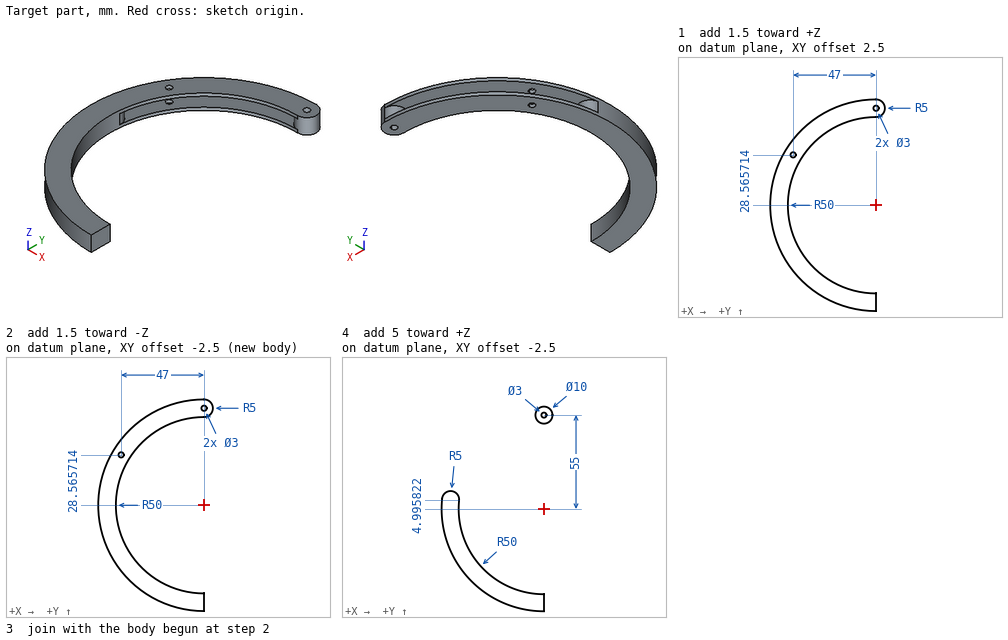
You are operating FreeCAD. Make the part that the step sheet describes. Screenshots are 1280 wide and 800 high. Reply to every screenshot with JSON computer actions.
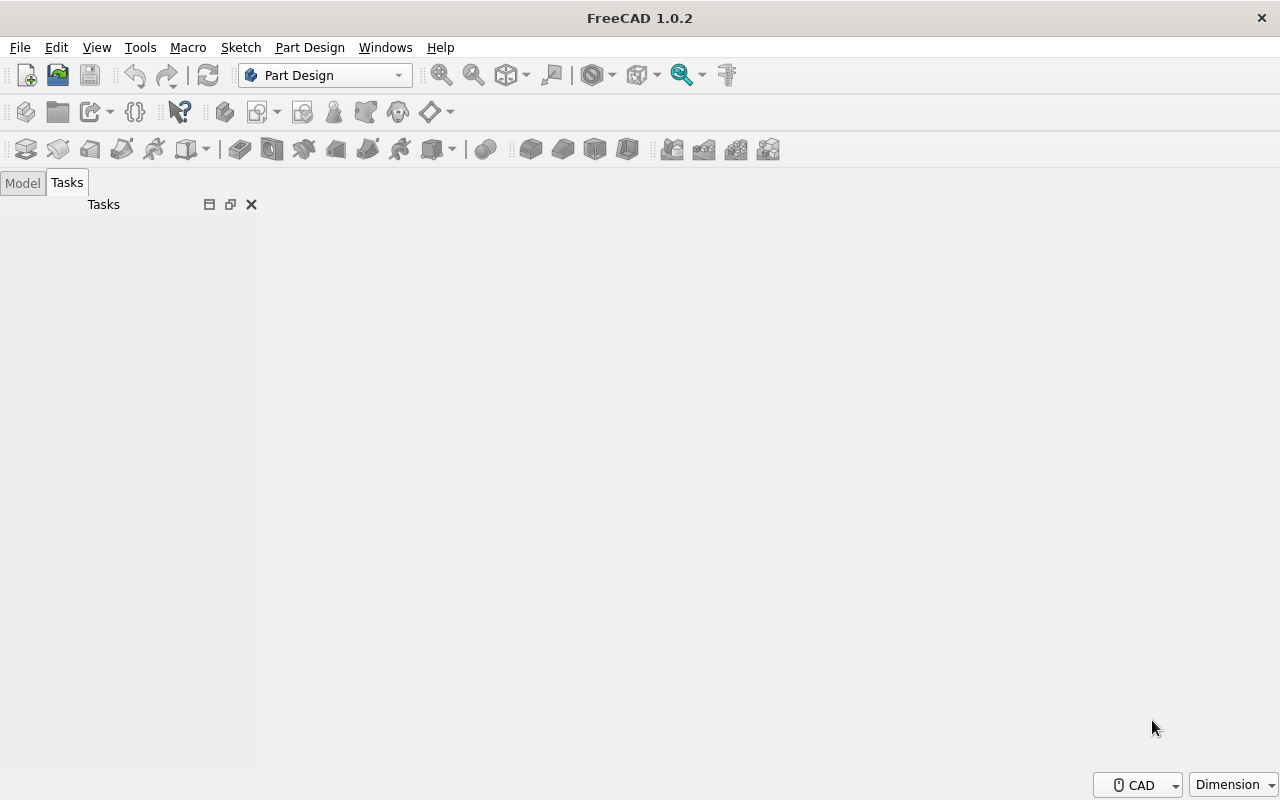
{"action": "left_click", "coordinate": [26, 76]}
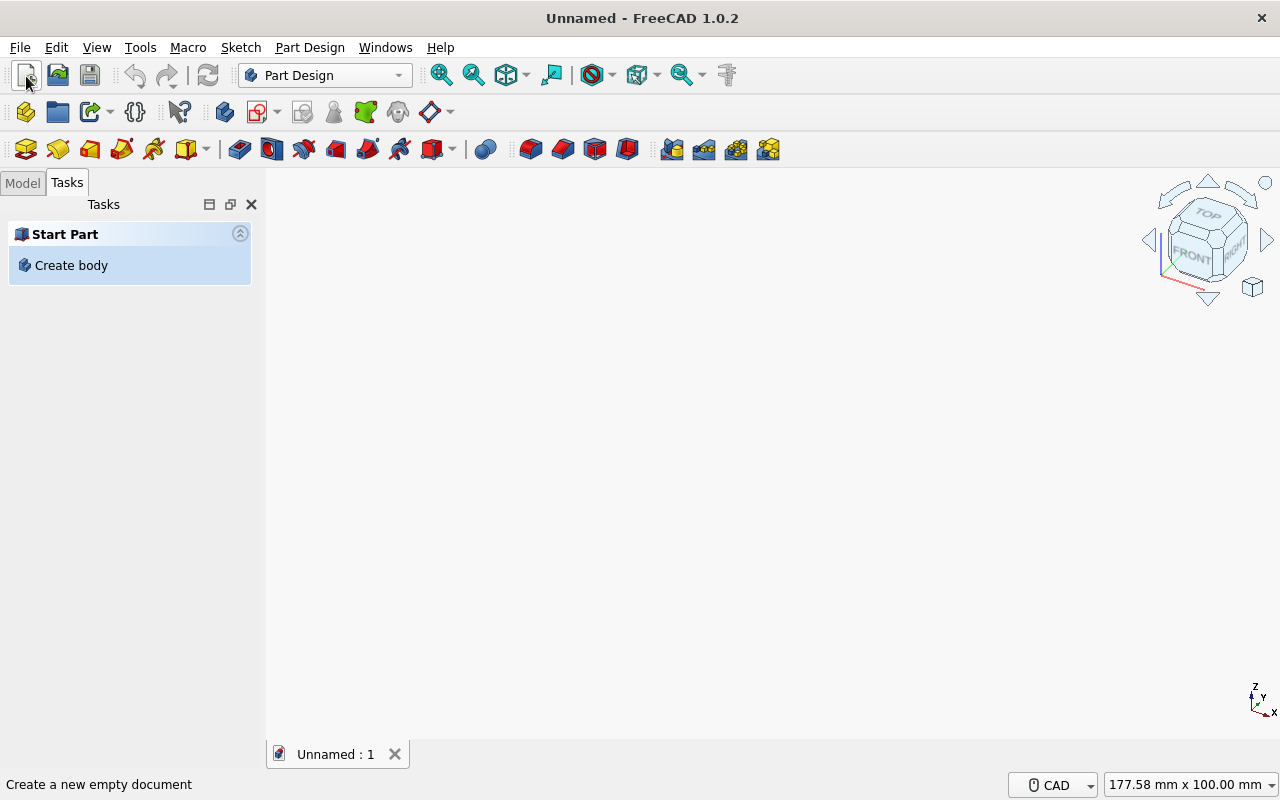
{"action": "left_click", "coordinate": [226, 112]}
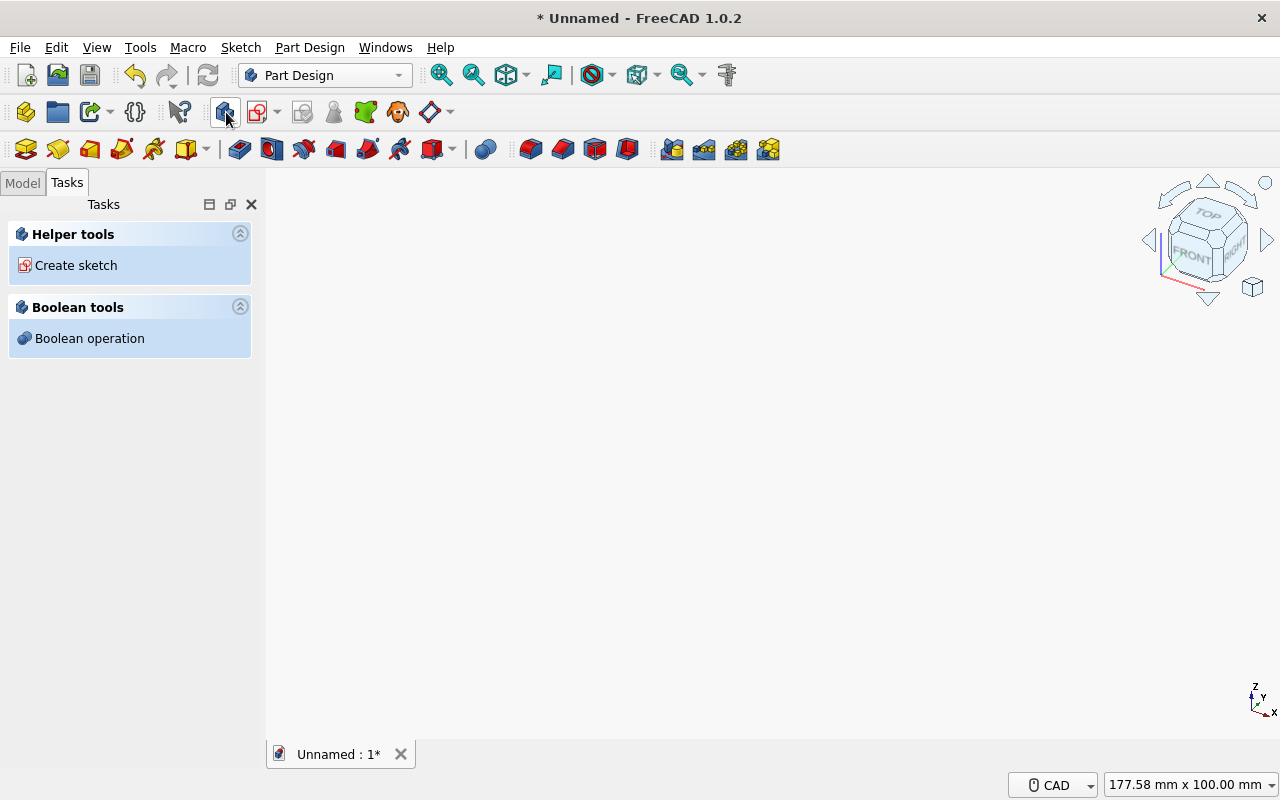
{"action": "left_click", "coordinate": [23, 182]}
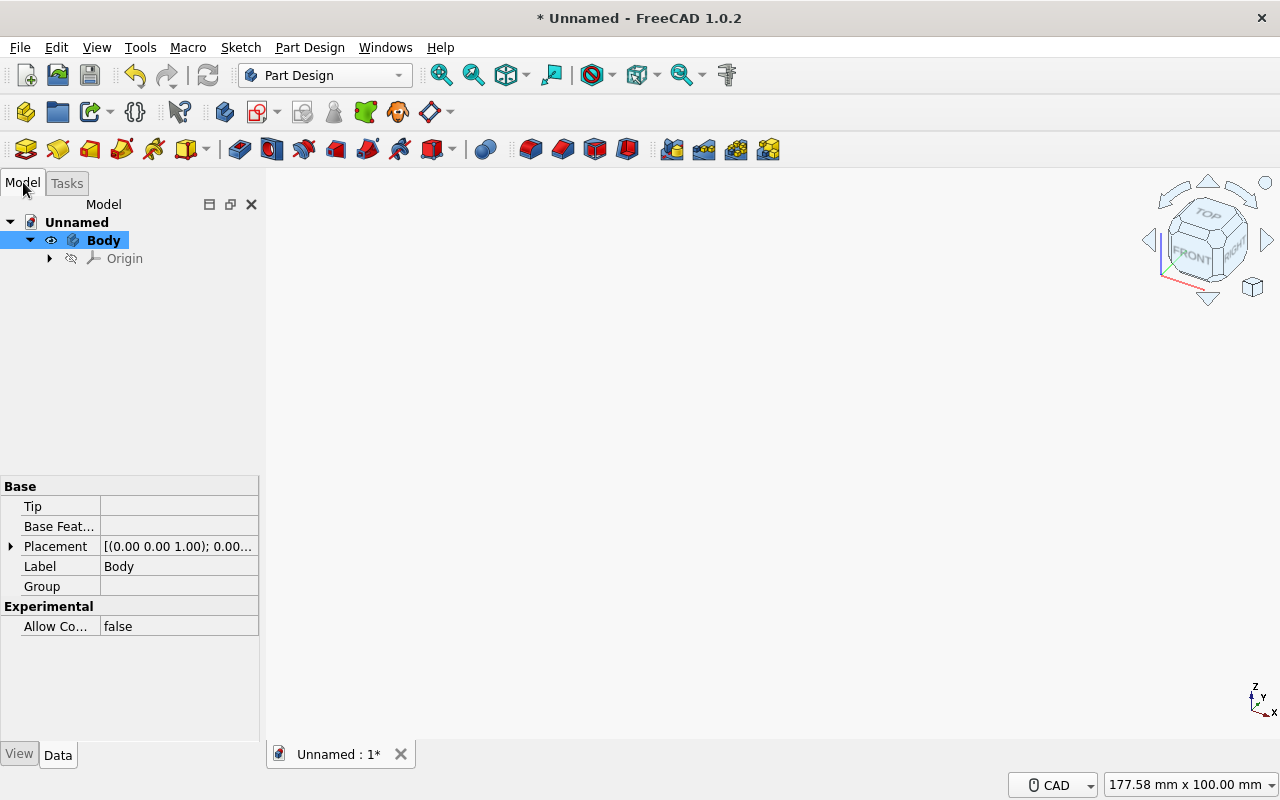
{"action": "left_click", "coordinate": [50, 258]}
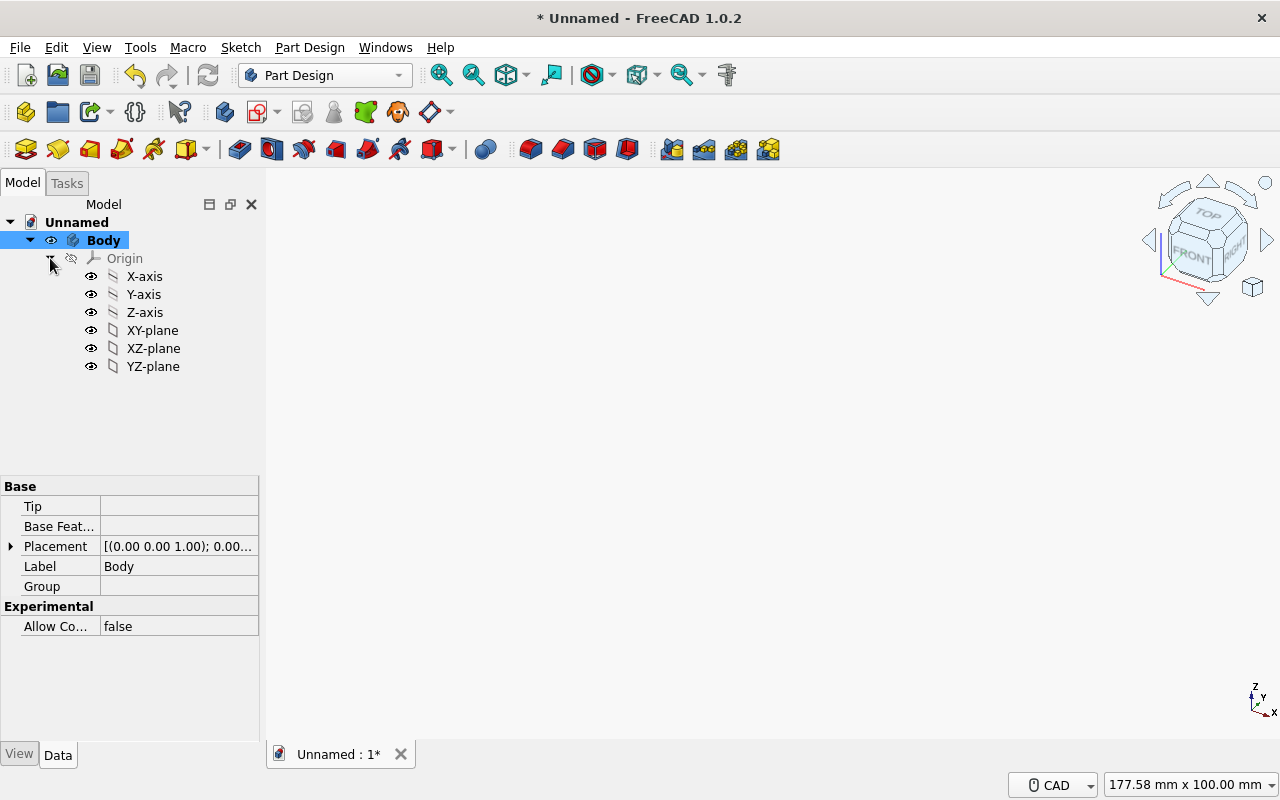
{"action": "left_click", "coordinate": [136, 330]}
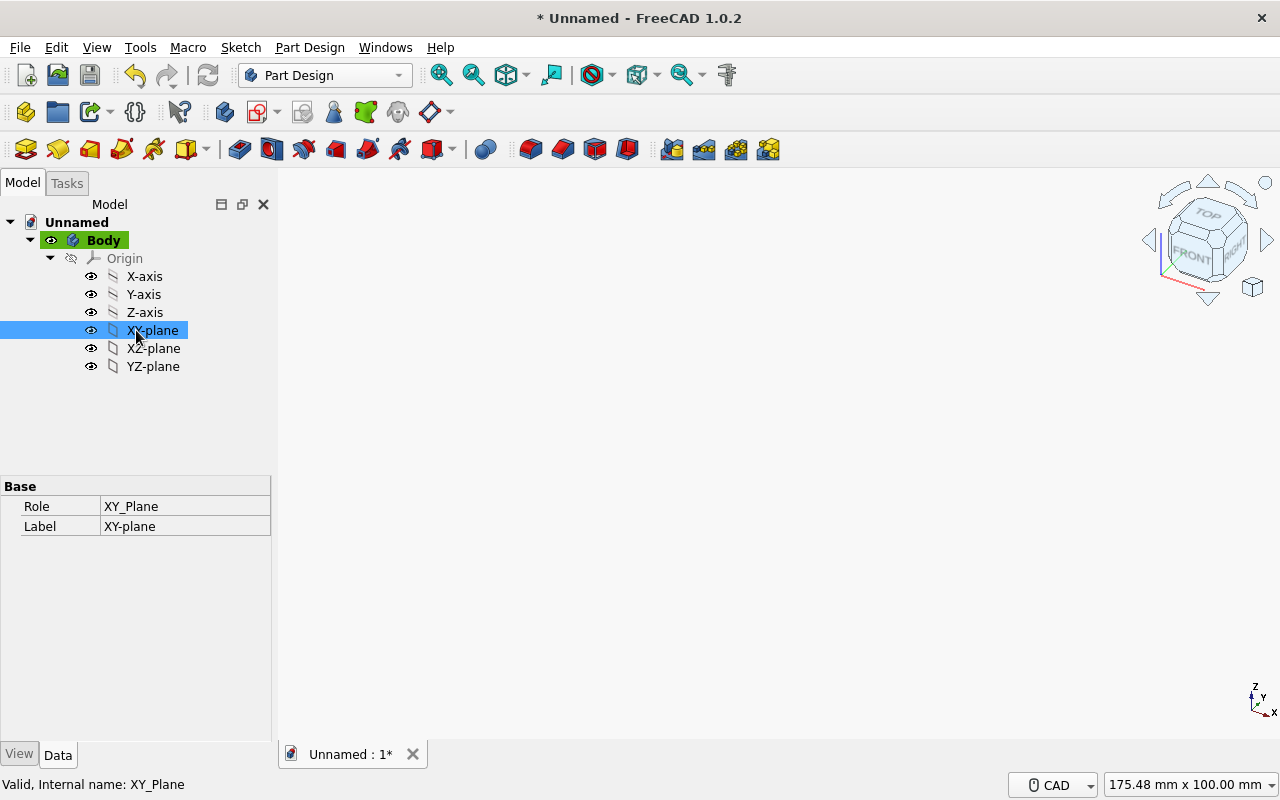
{"action": "left_click", "coordinate": [430, 112]}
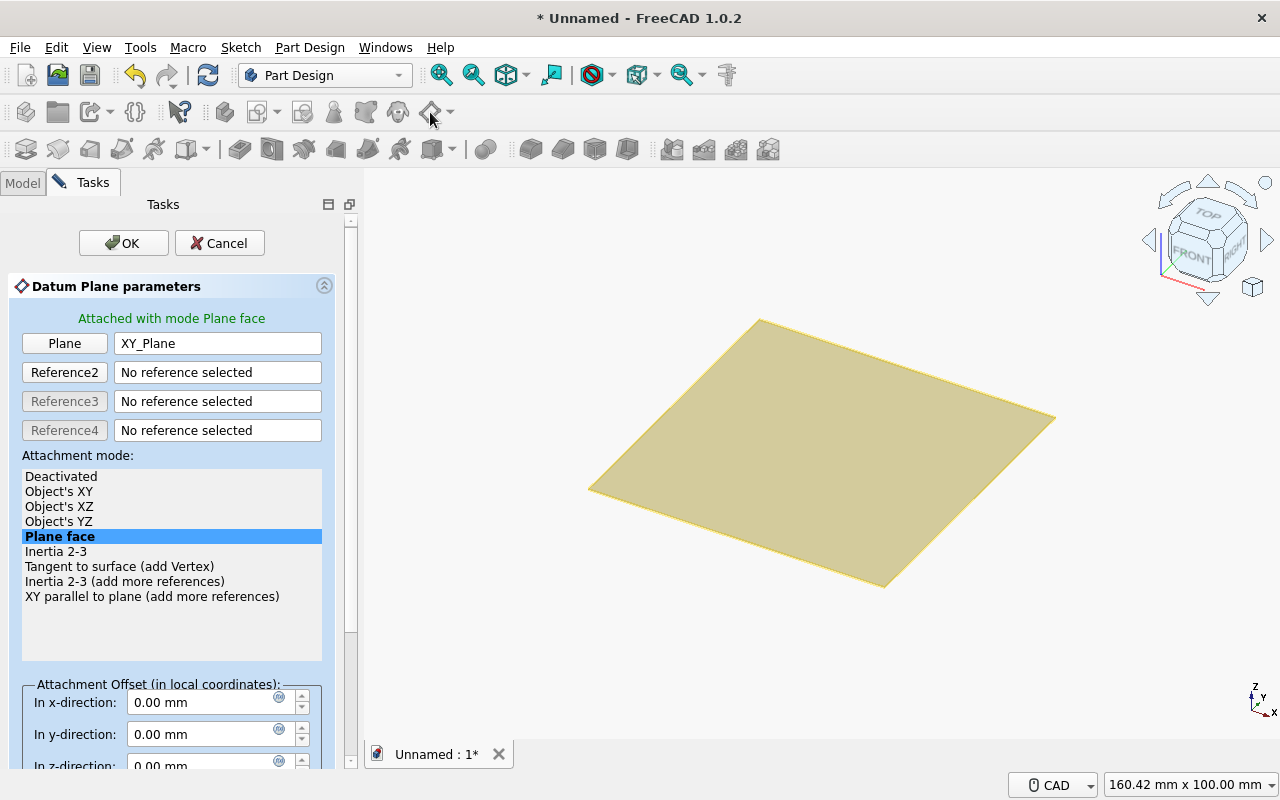
{"action": "scroll", "coordinate": [351, 491], "scroll_direction": "down", "scroll_amount": 2}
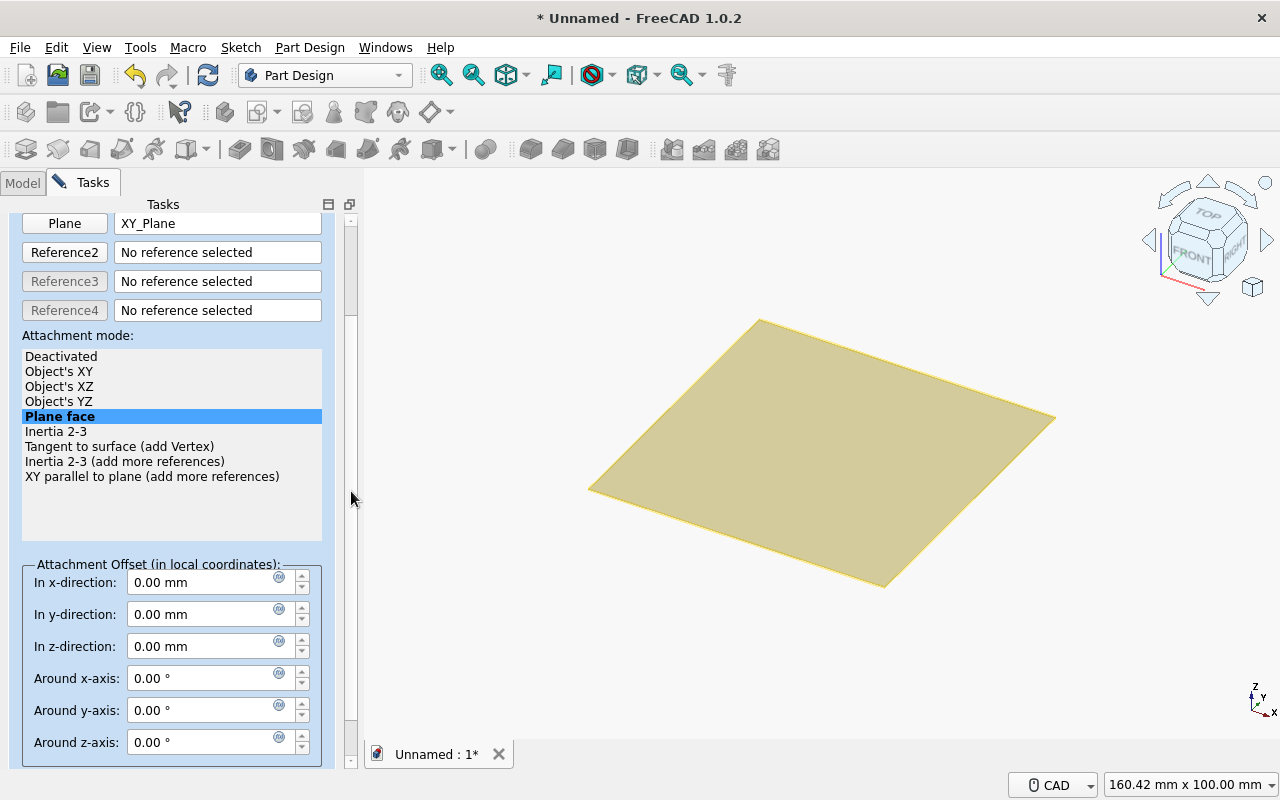
{"action": "triple_click", "coordinate": [210, 646]}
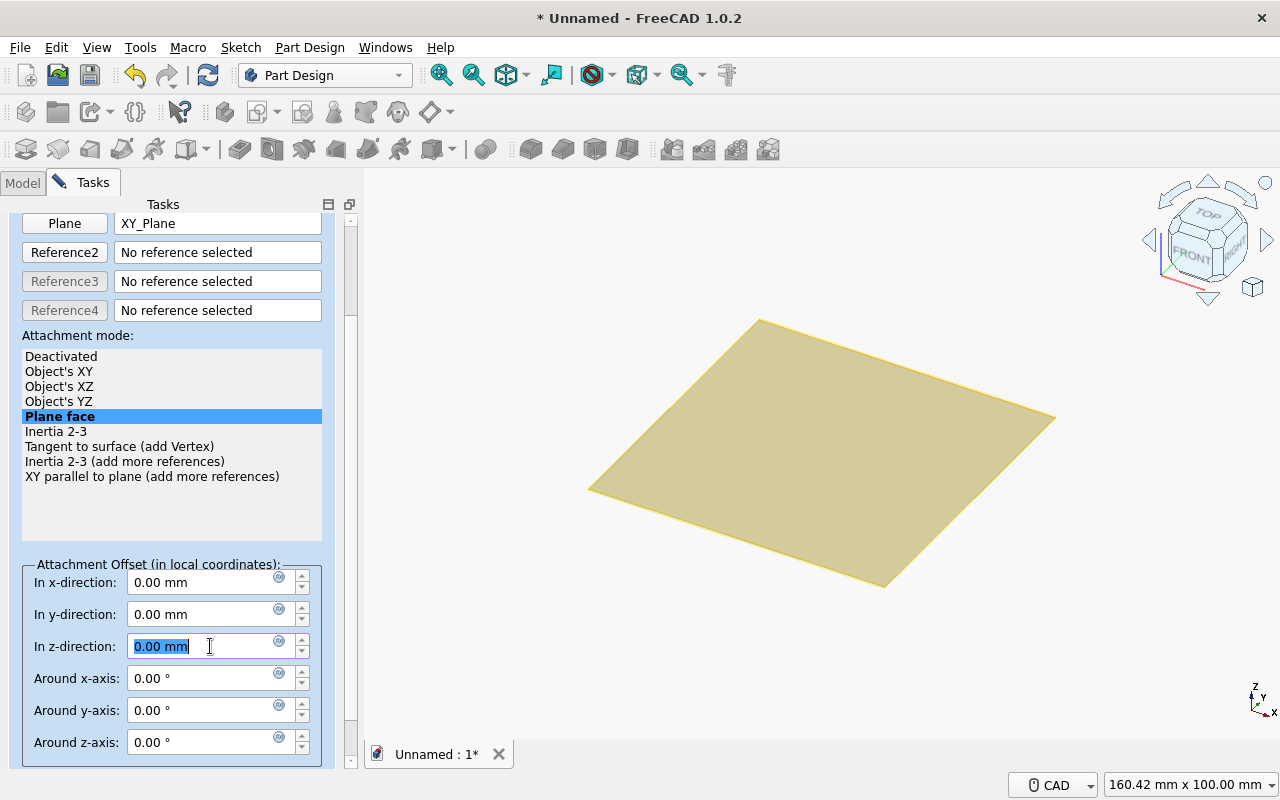
{"action": "type", "text": "2.5"}
{"action": "key", "text": "Tab"}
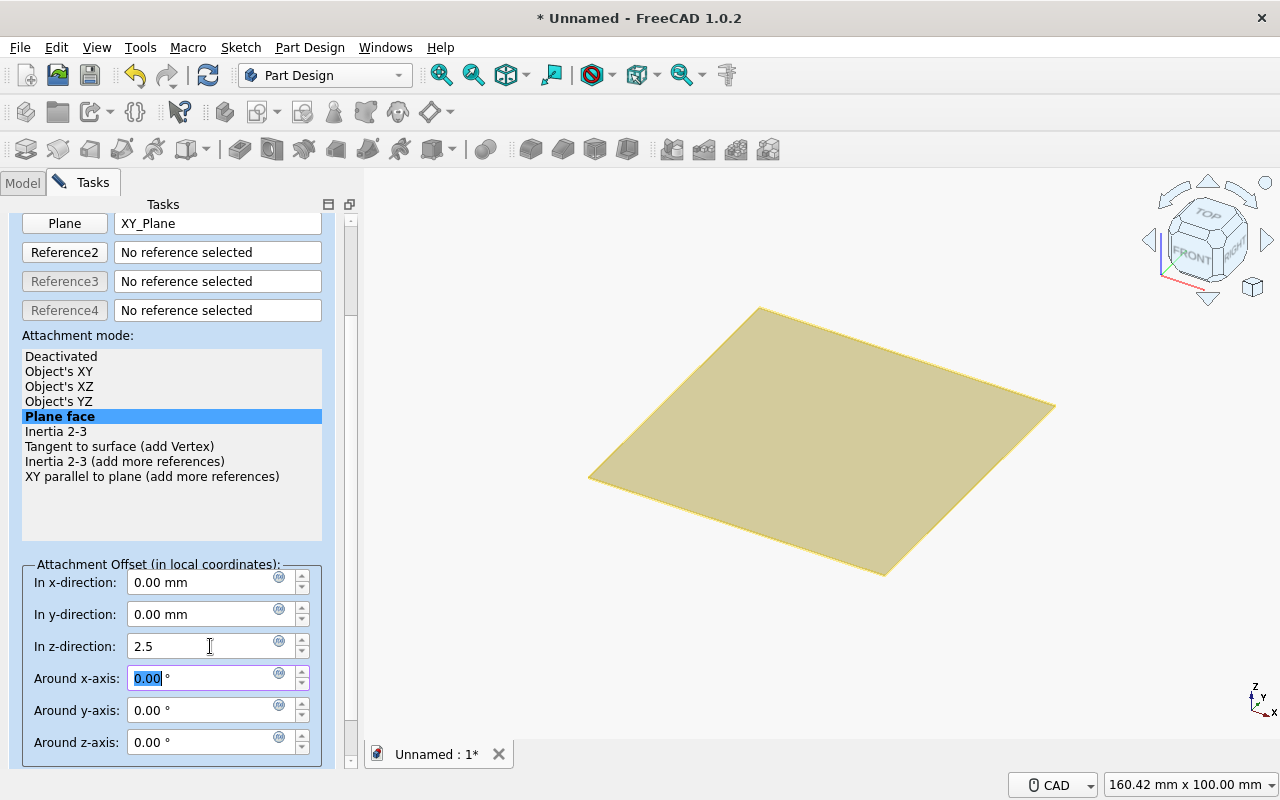
{"action": "scroll", "coordinate": [351, 491], "scroll_direction": "up", "scroll_amount": 3}